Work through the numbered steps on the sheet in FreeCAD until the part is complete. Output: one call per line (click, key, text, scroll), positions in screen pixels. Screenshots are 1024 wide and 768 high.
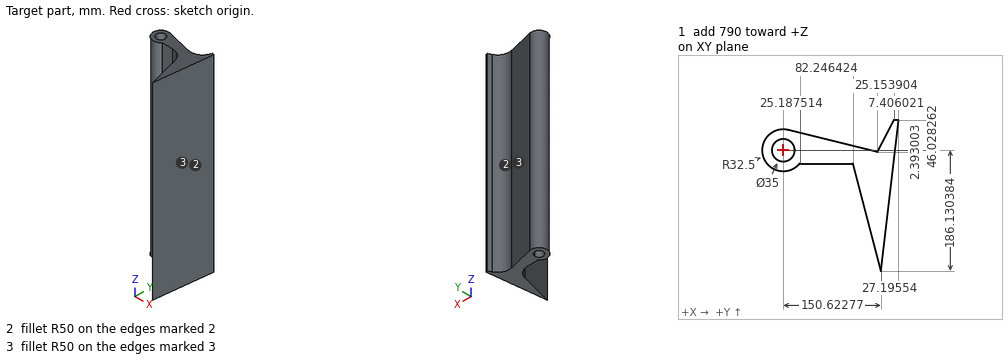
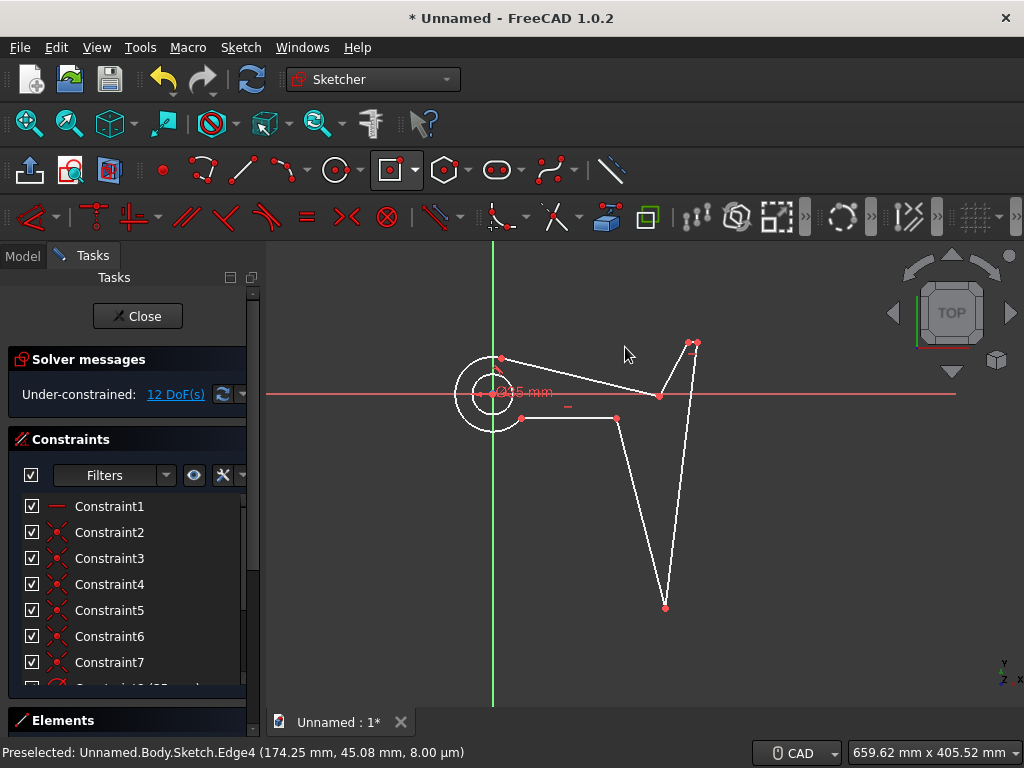
scroll(493, 394, up, 4)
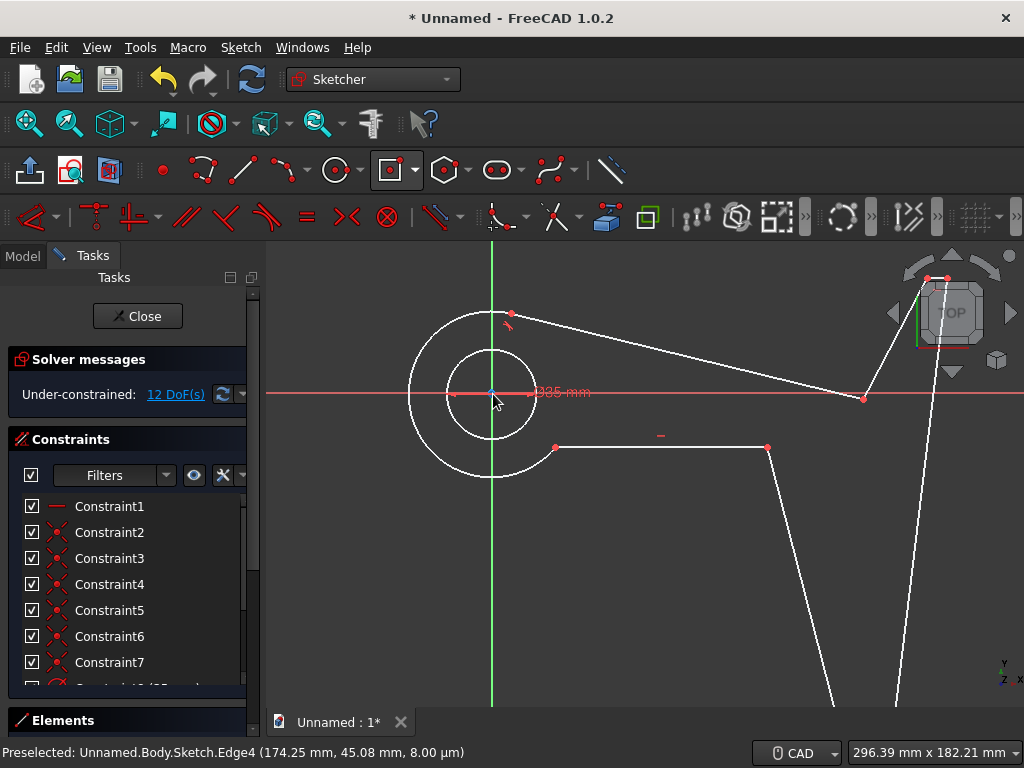
drag(482, 383, 502, 404)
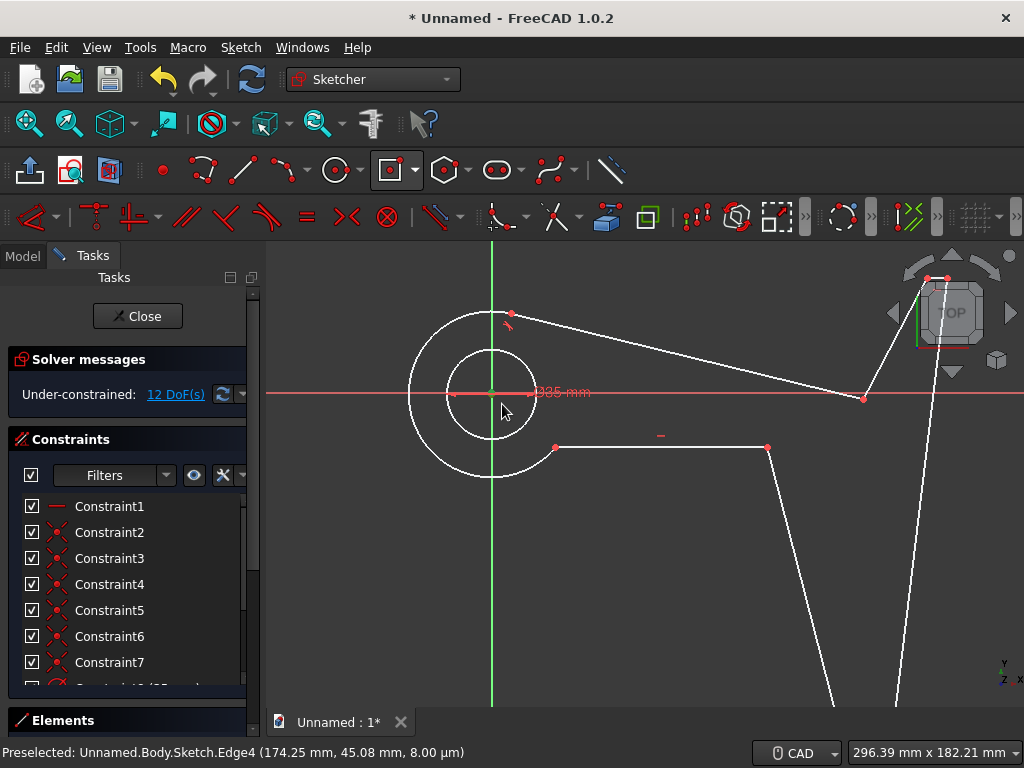
key(c)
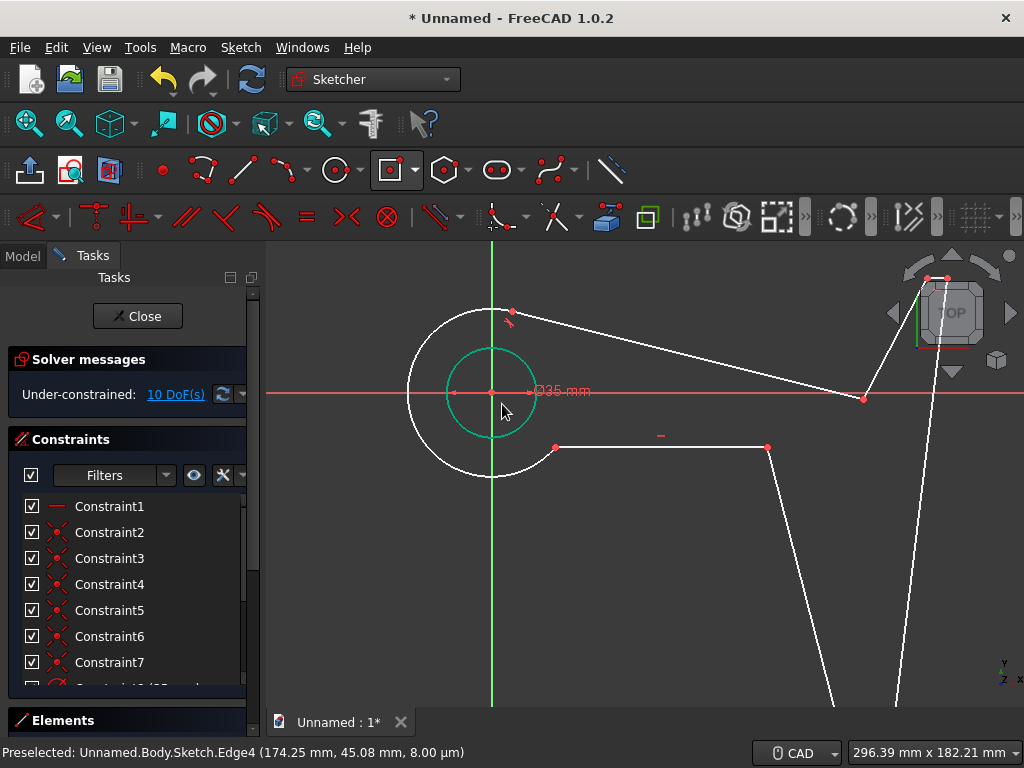
key(d)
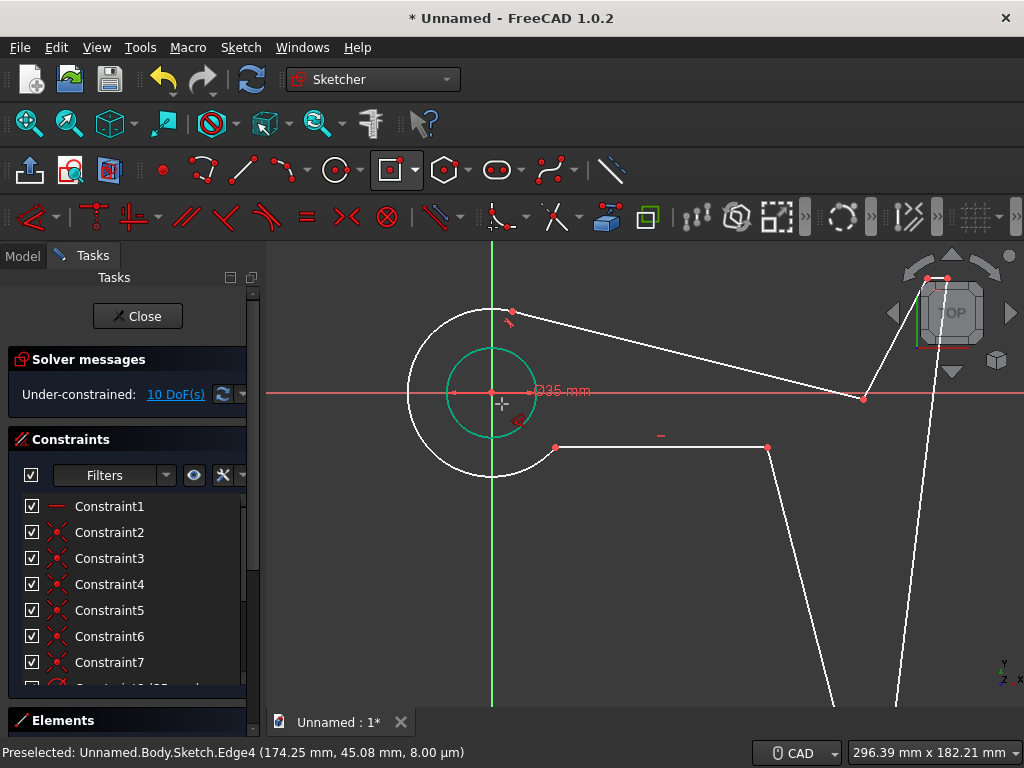
click(420, 350)
click(393, 334)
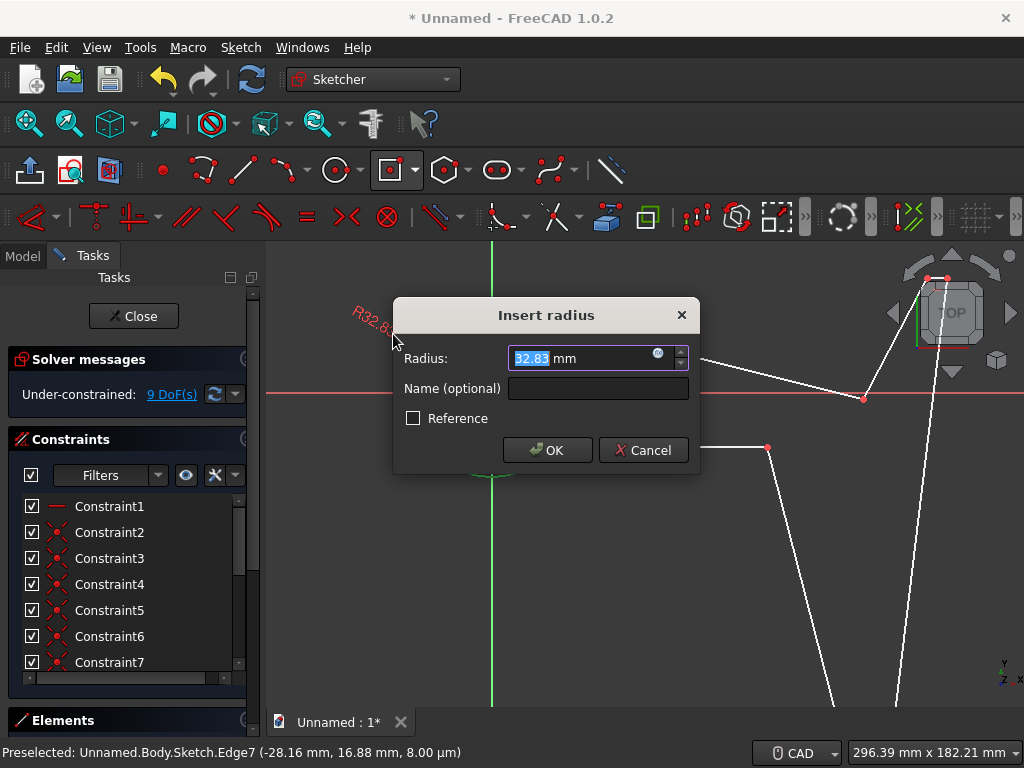
text(32.5)
key(Return)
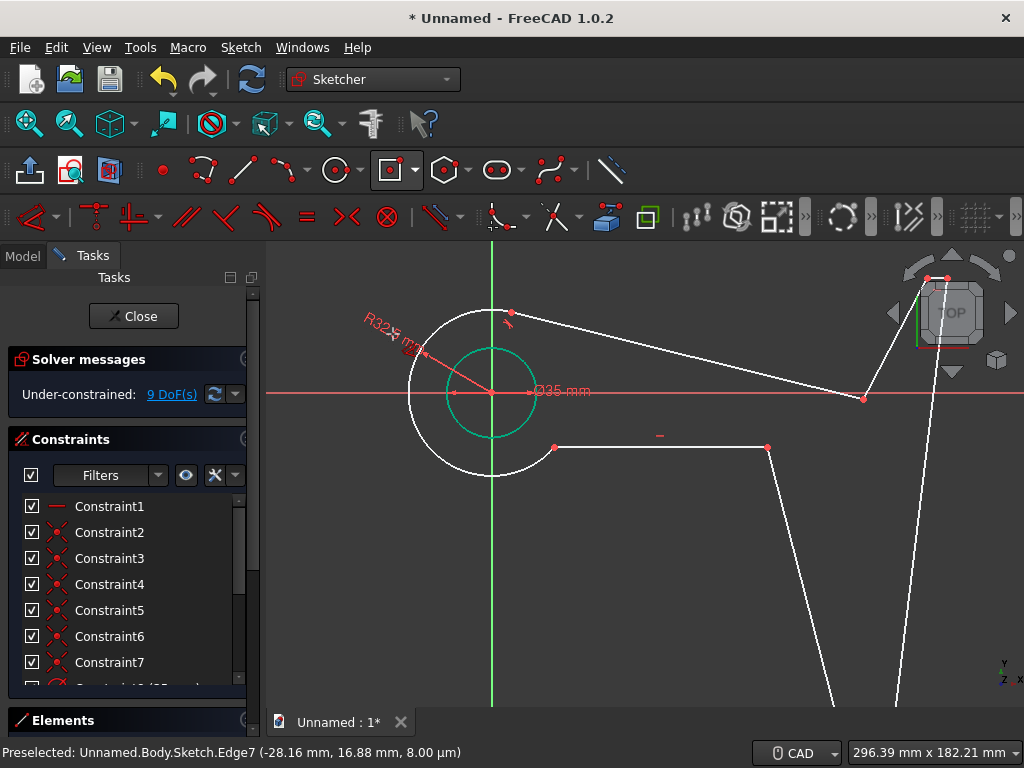
scroll(492, 394, down, 4)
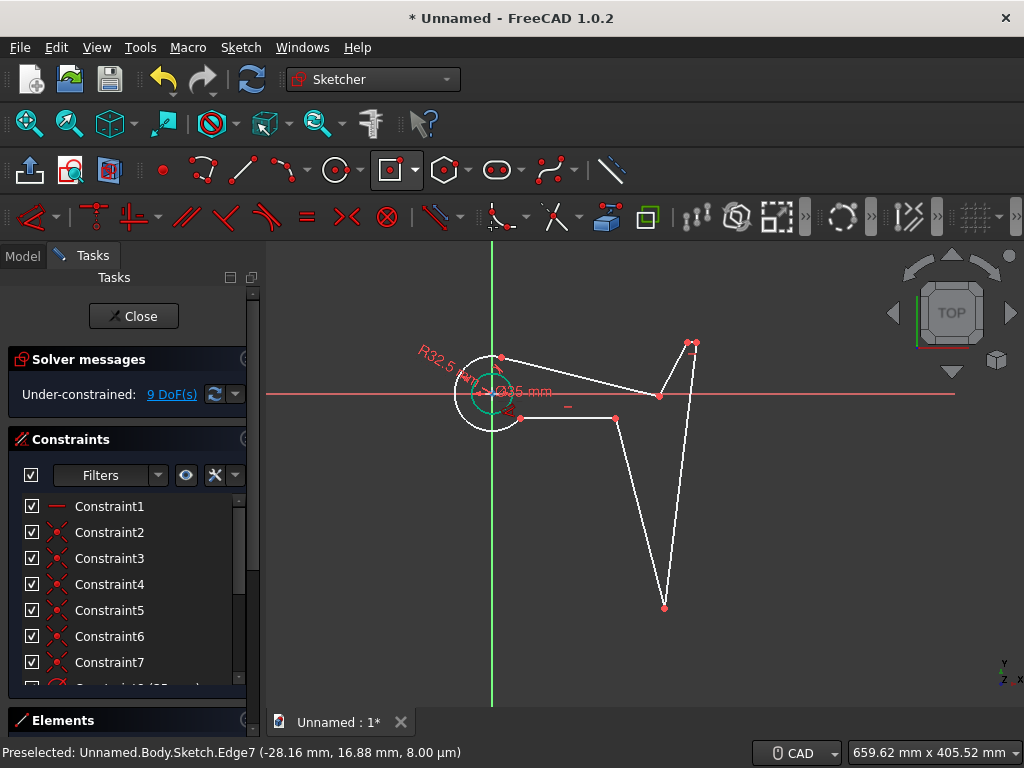
scroll(692, 342, up, 8)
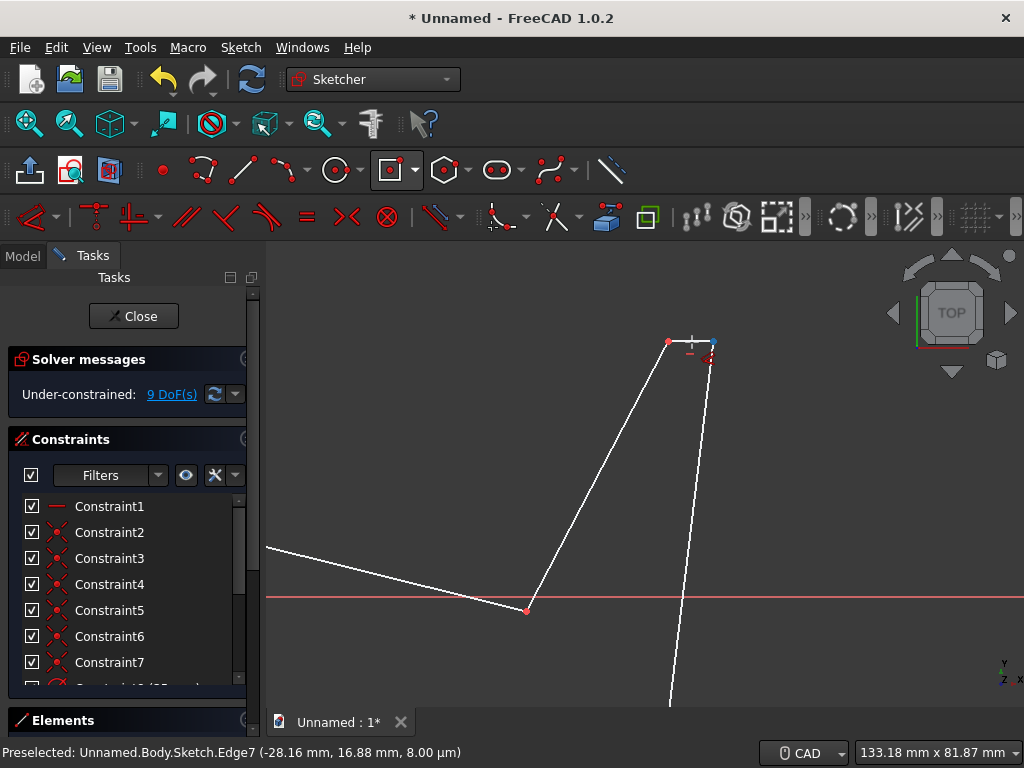
click(691, 341)
click(691, 307)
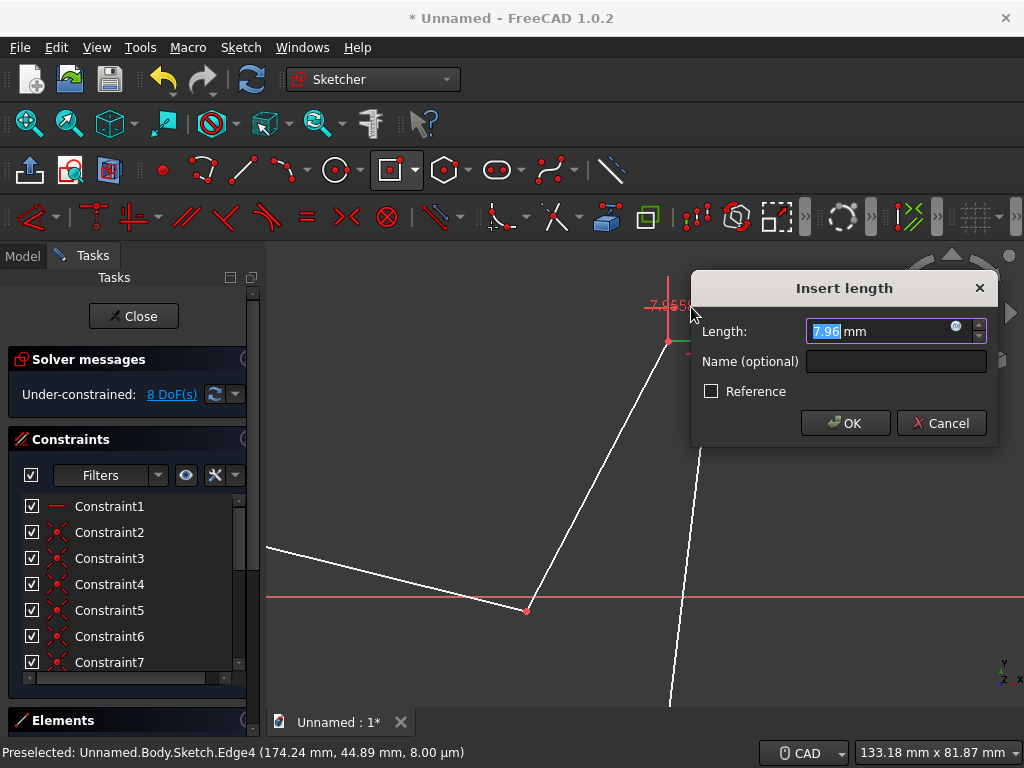
text(7.406021)
key(Return)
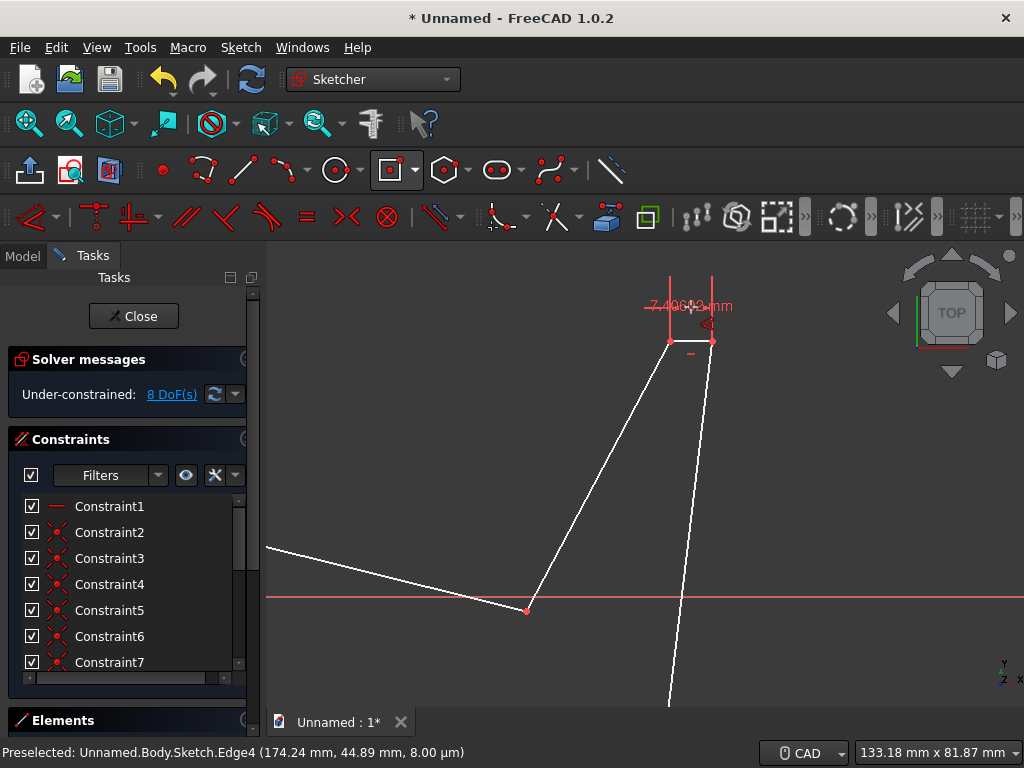
scroll(693, 342, down, 8)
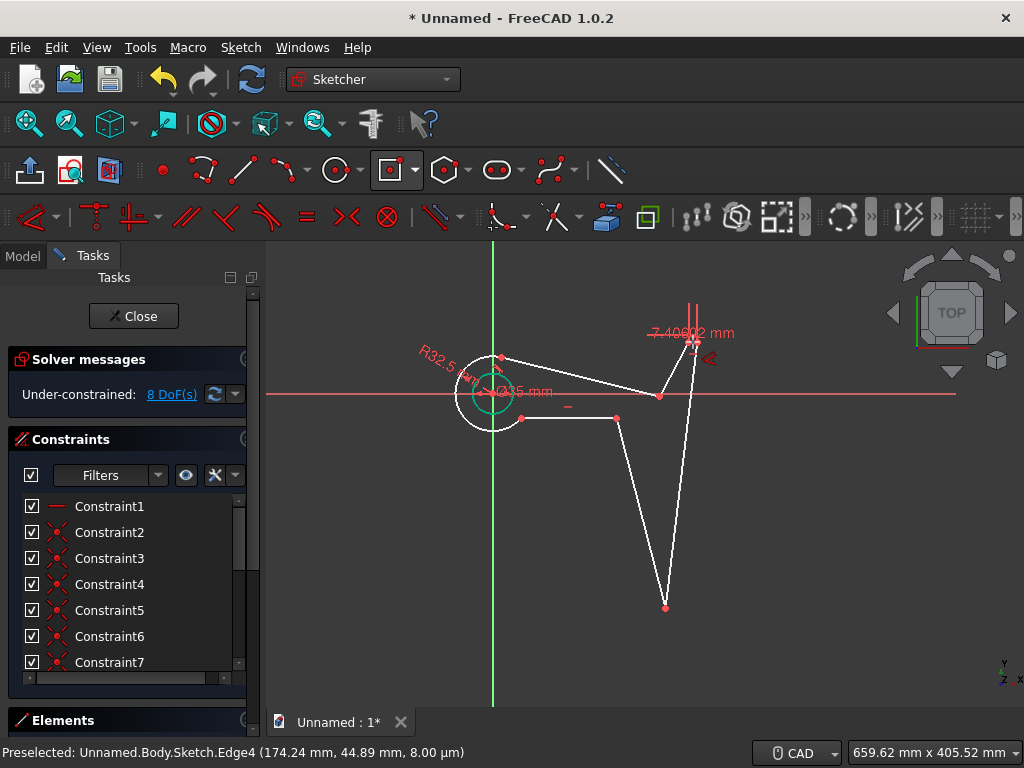
click(550, 418)
click(569, 452)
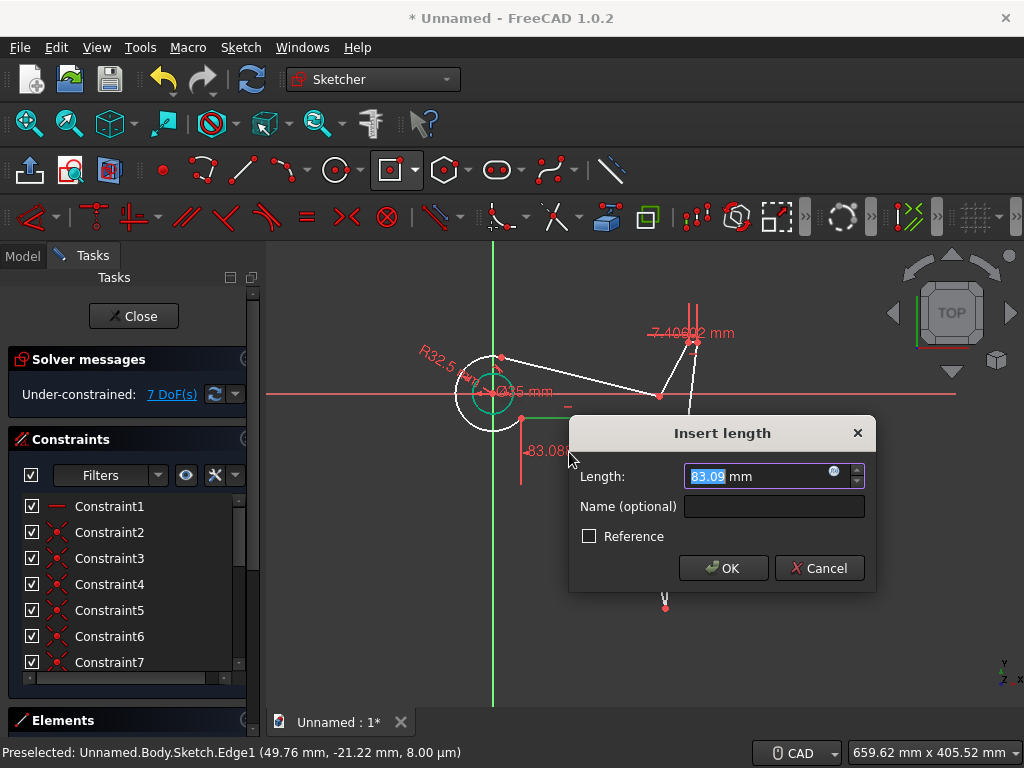
text(82.246424)
key(Return)